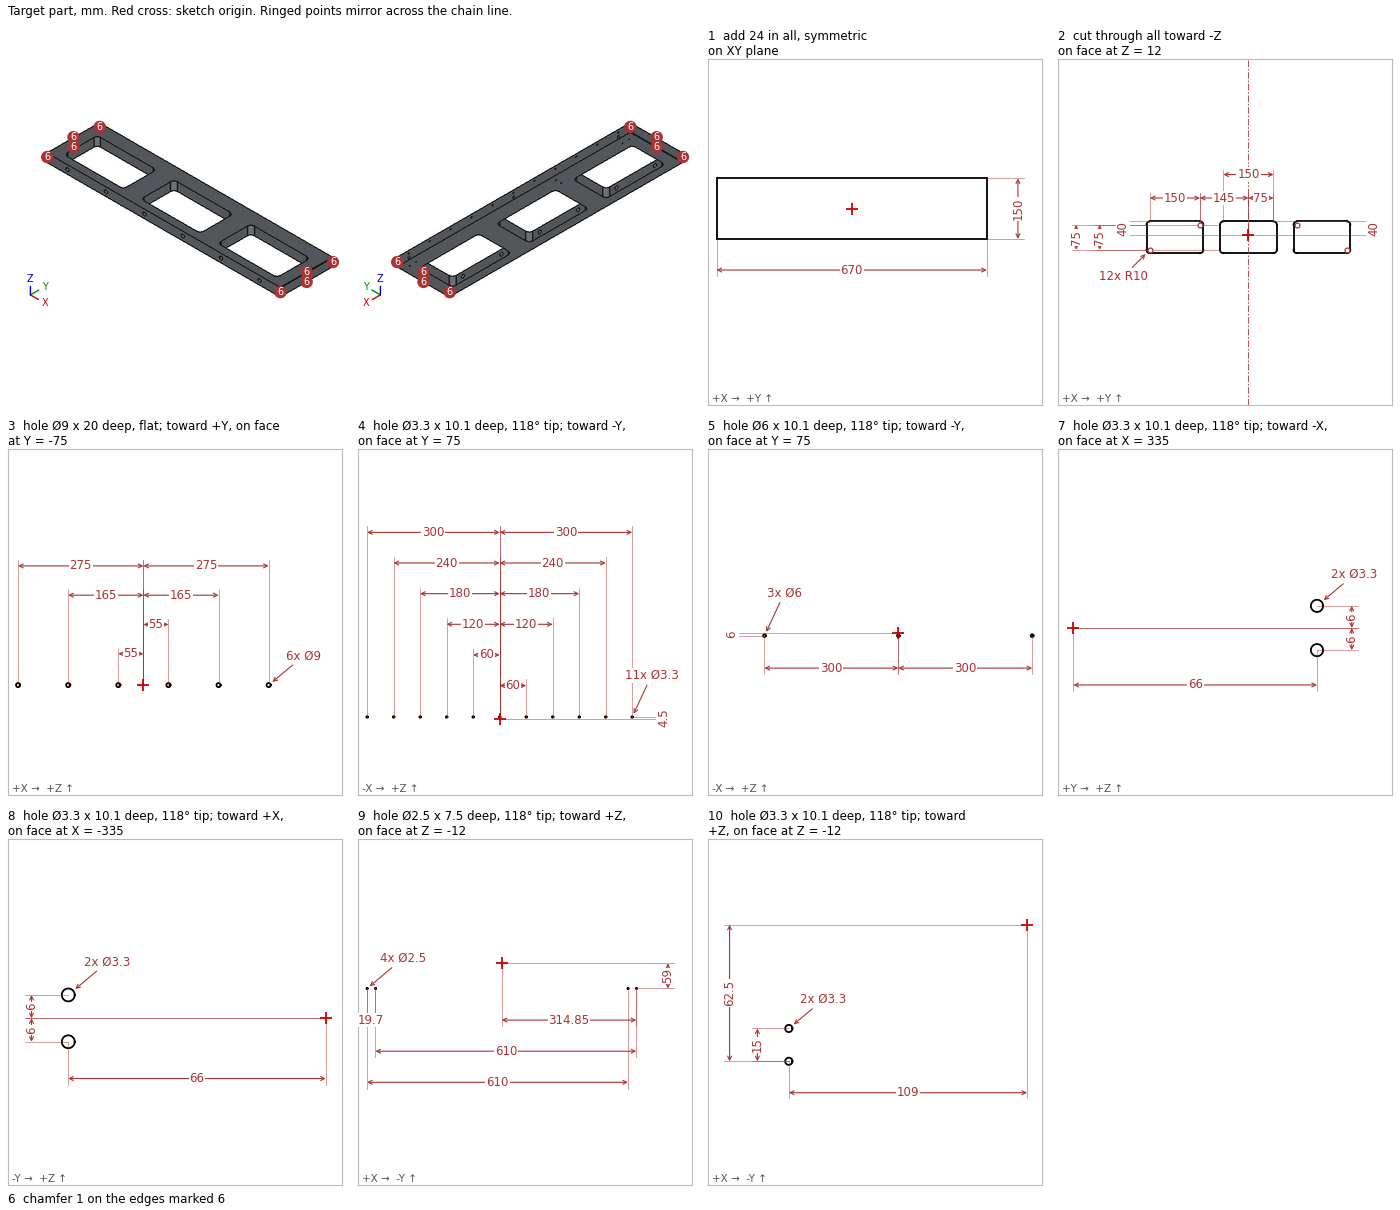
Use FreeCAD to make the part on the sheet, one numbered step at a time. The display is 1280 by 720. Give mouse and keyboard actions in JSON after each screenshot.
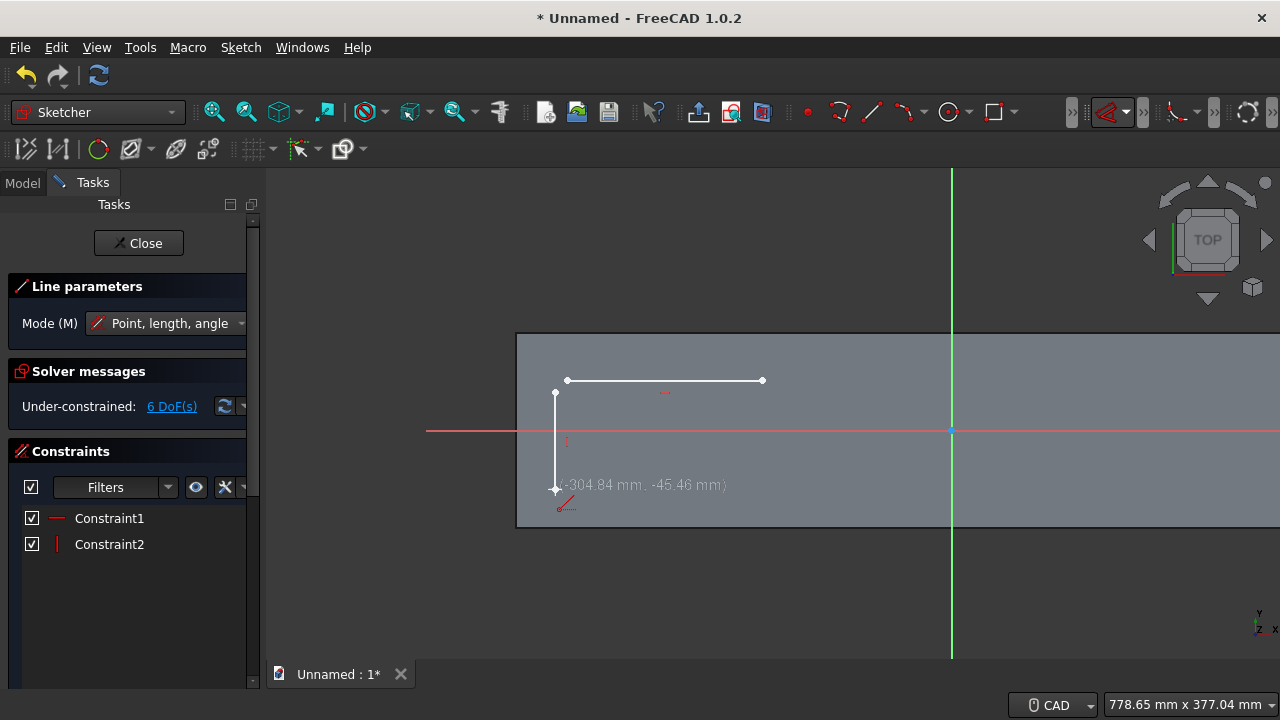
{"action": "left_click", "coordinate": [568, 502]}
{"action": "left_click", "coordinate": [763, 502]}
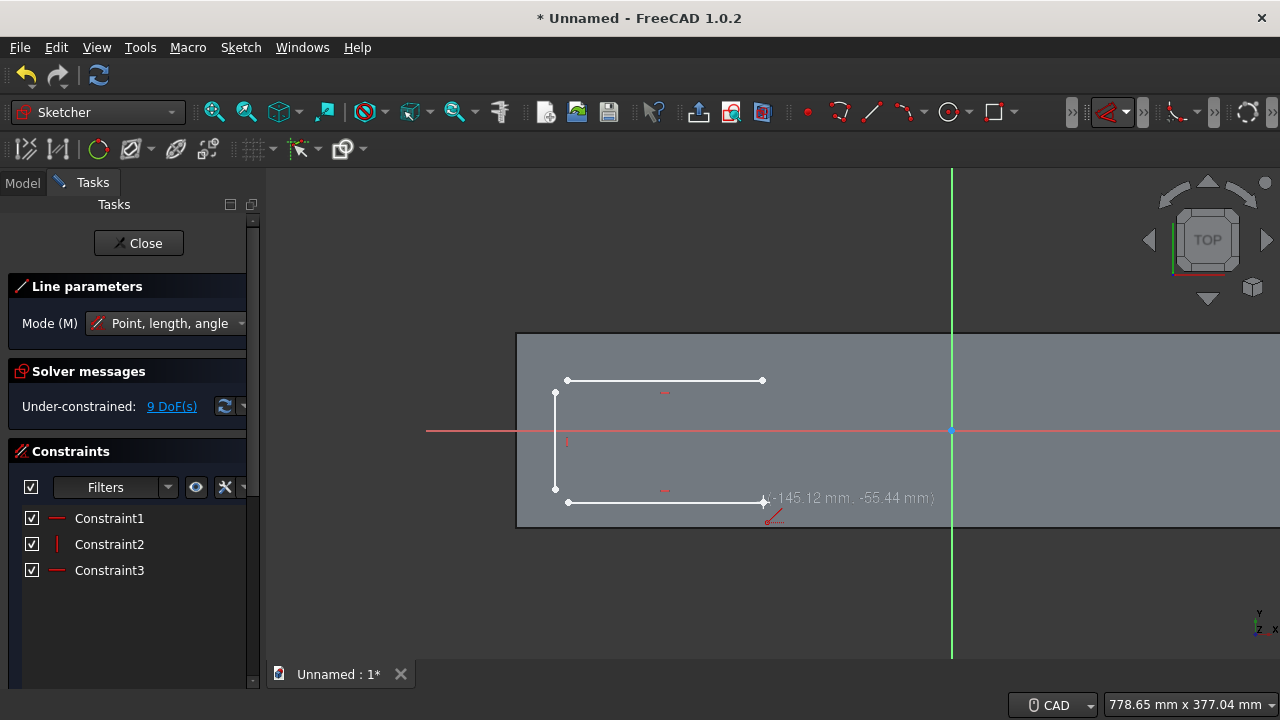
{"action": "left_click", "coordinate": [776, 489]}
{"action": "left_click", "coordinate": [776, 392]}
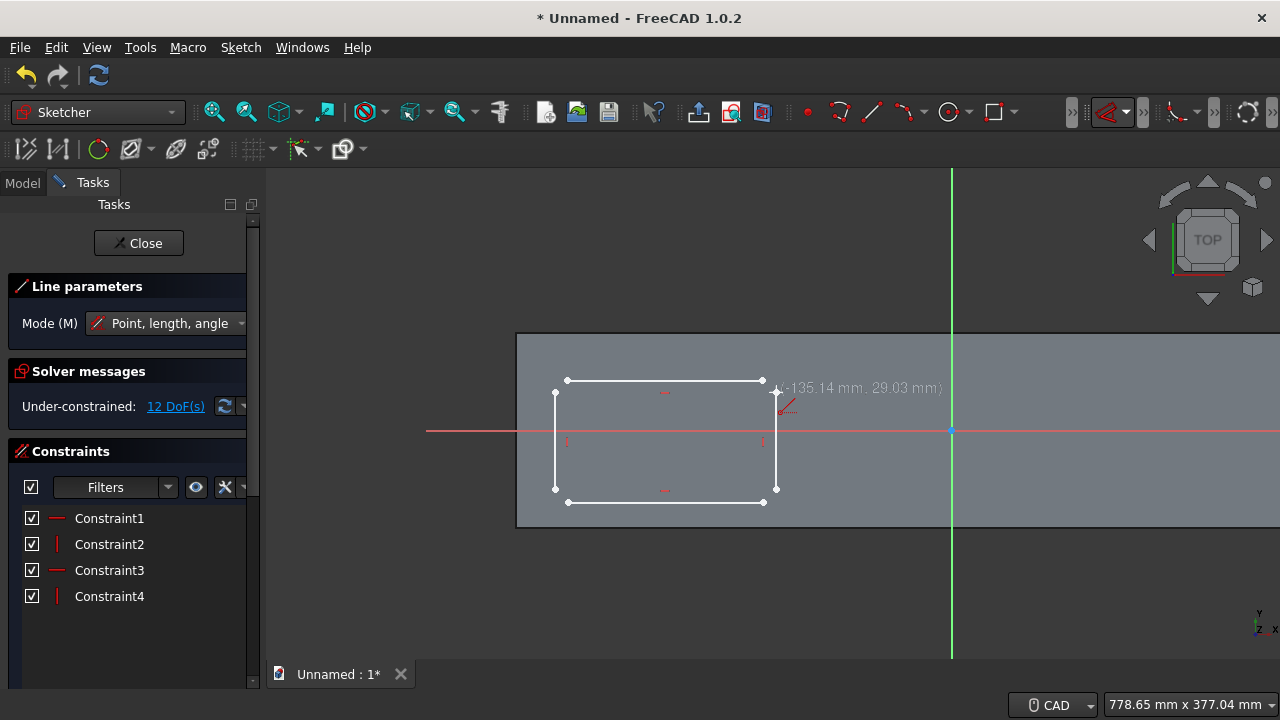
{"action": "left_click", "coordinate": [904, 112]}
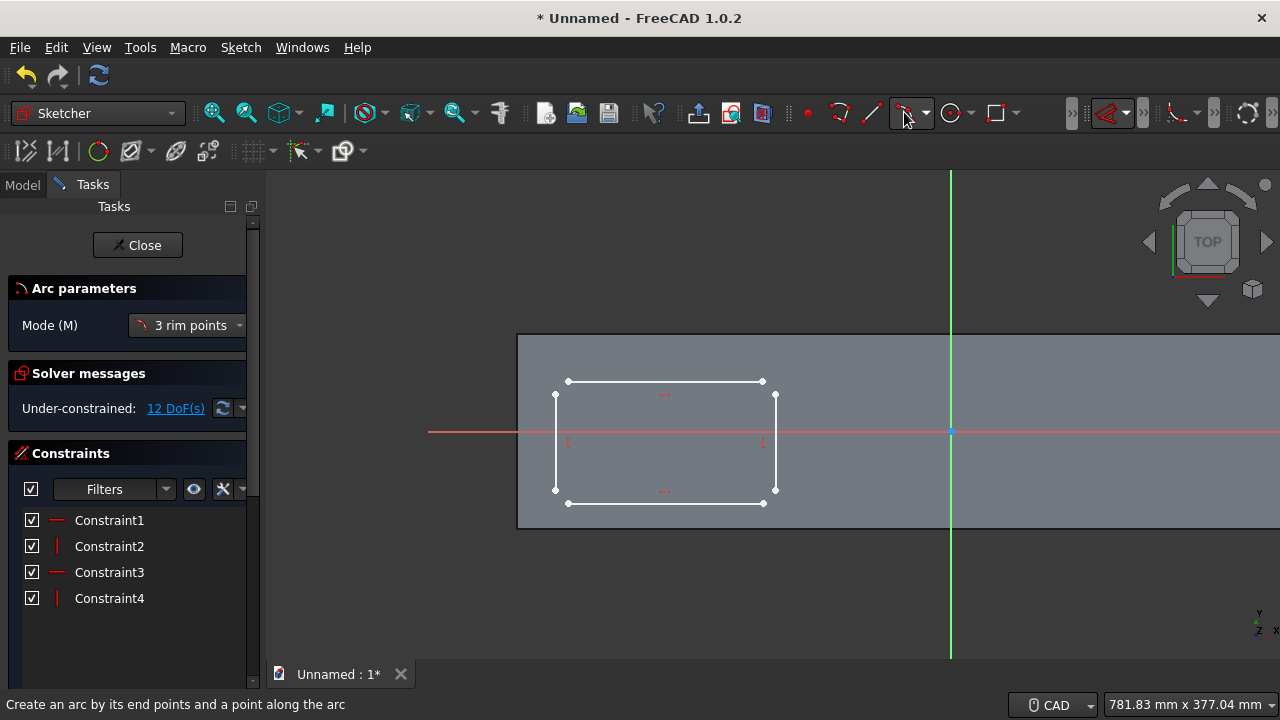
{"action": "left_click", "coordinate": [568, 382]}
{"action": "left_click", "coordinate": [556, 394]}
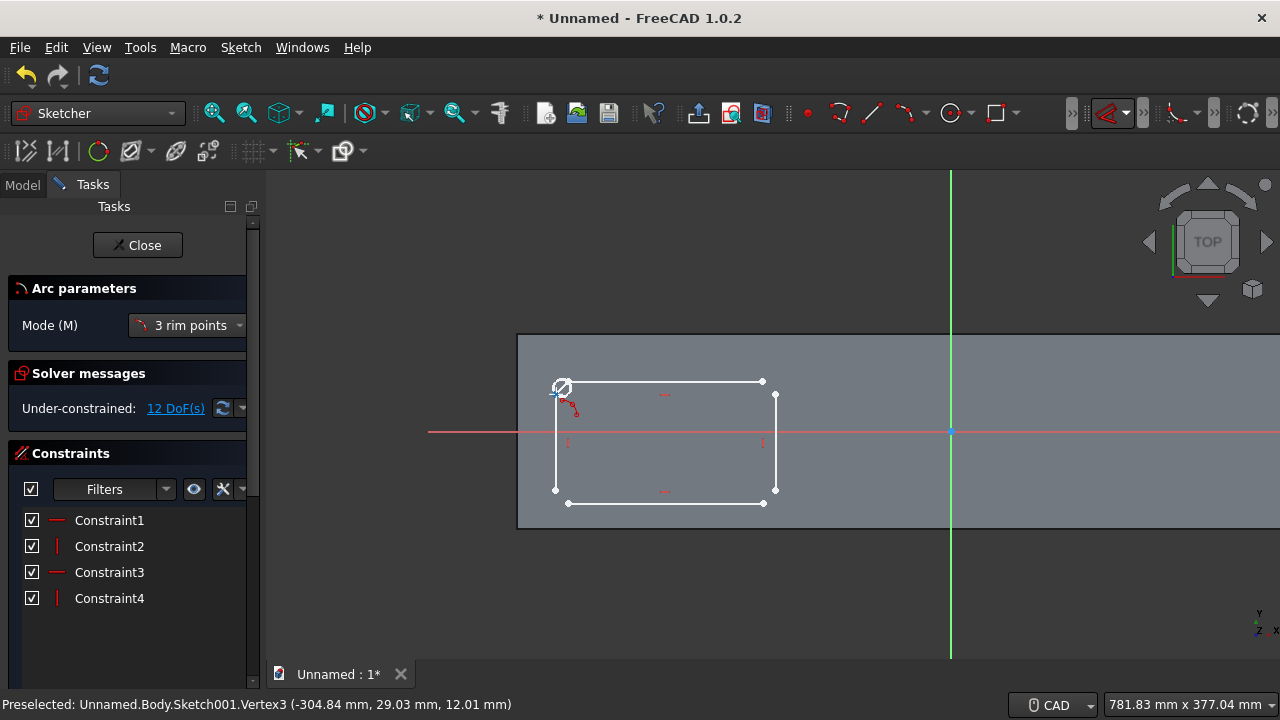
{"action": "scroll", "coordinate": [559, 384], "scroll_direction": "up", "scroll_amount": 8}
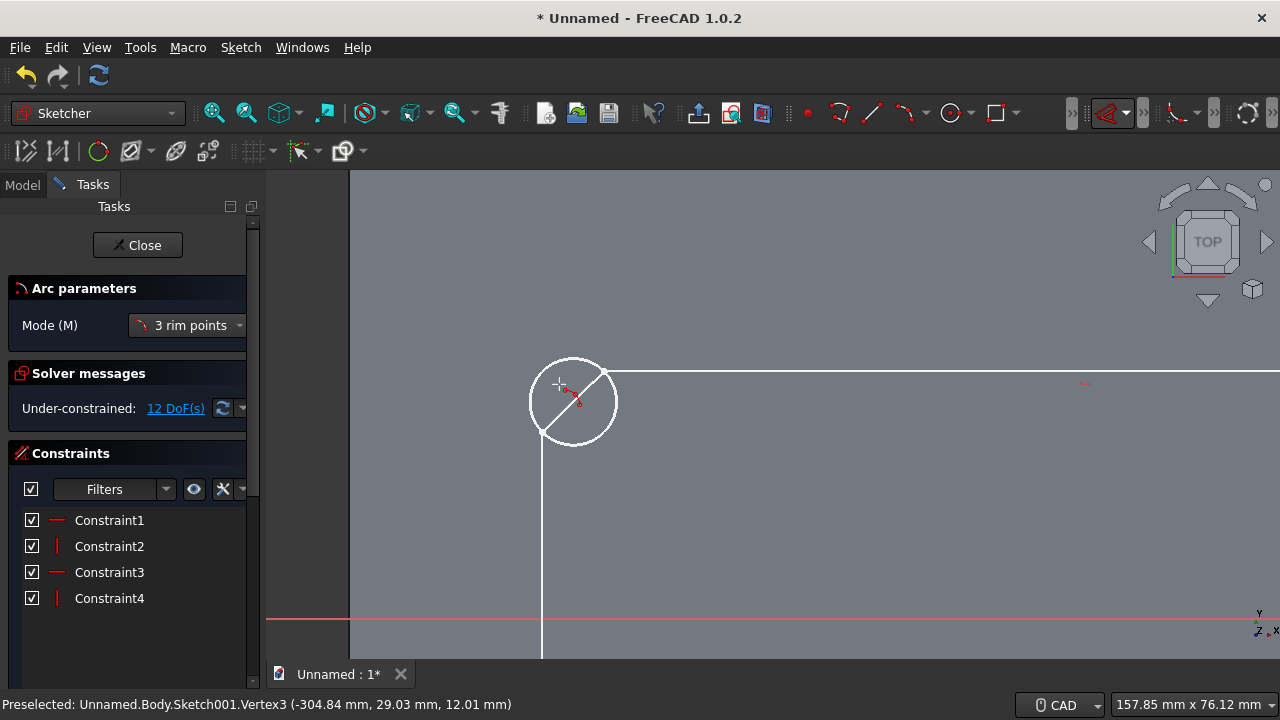
{"action": "left_click", "coordinate": [560, 381]}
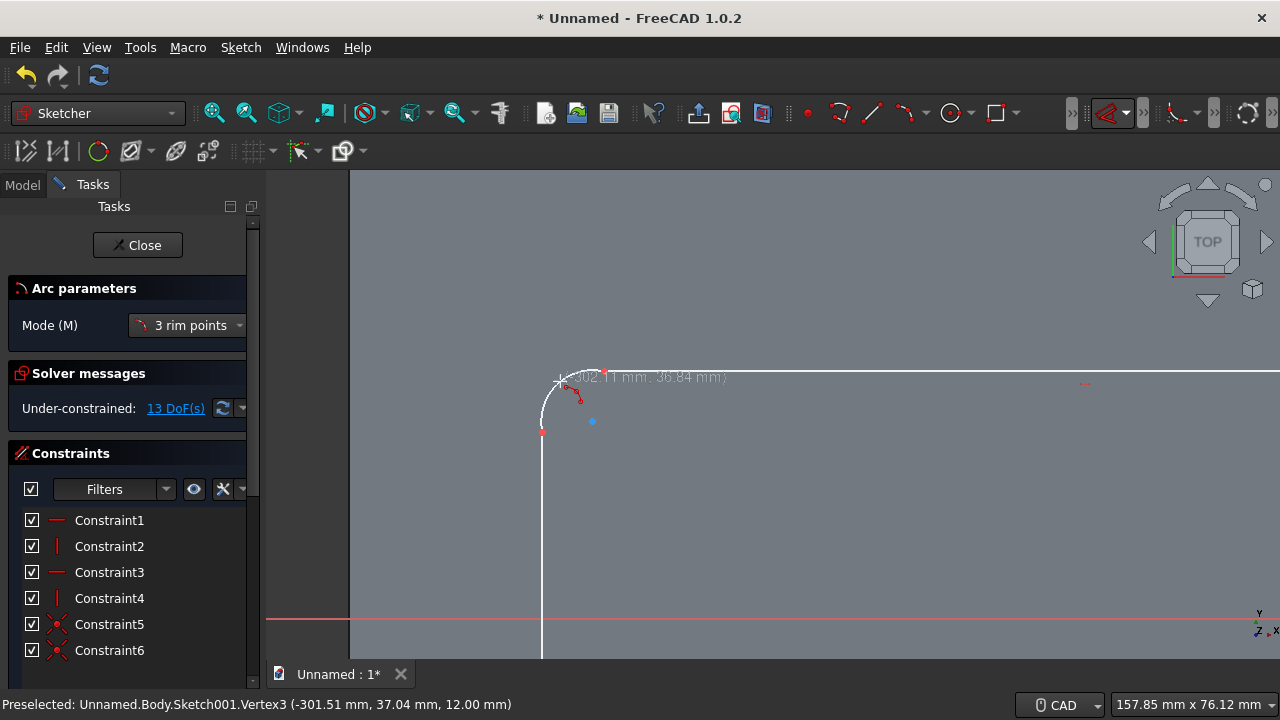
{"action": "scroll", "coordinate": [423, 375], "scroll_direction": "down", "scroll_amount": 10}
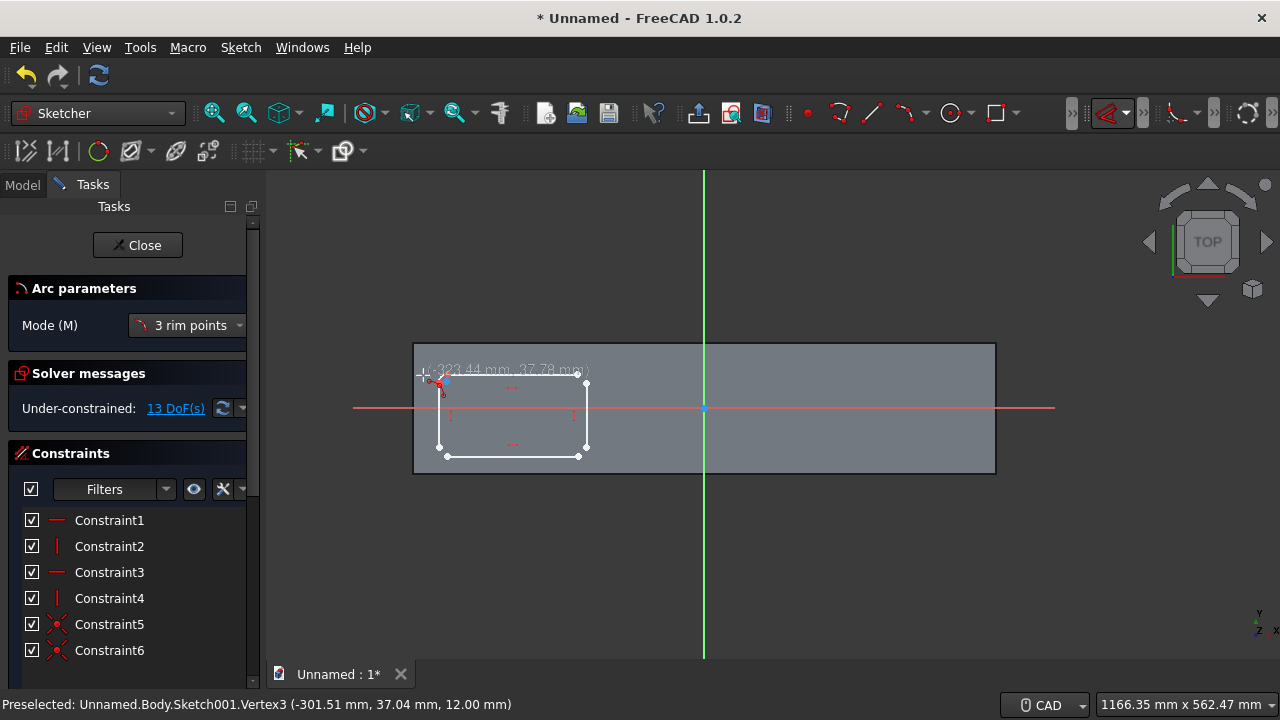
{"action": "scroll", "coordinate": [439, 447], "scroll_direction": "up", "scroll_amount": 2}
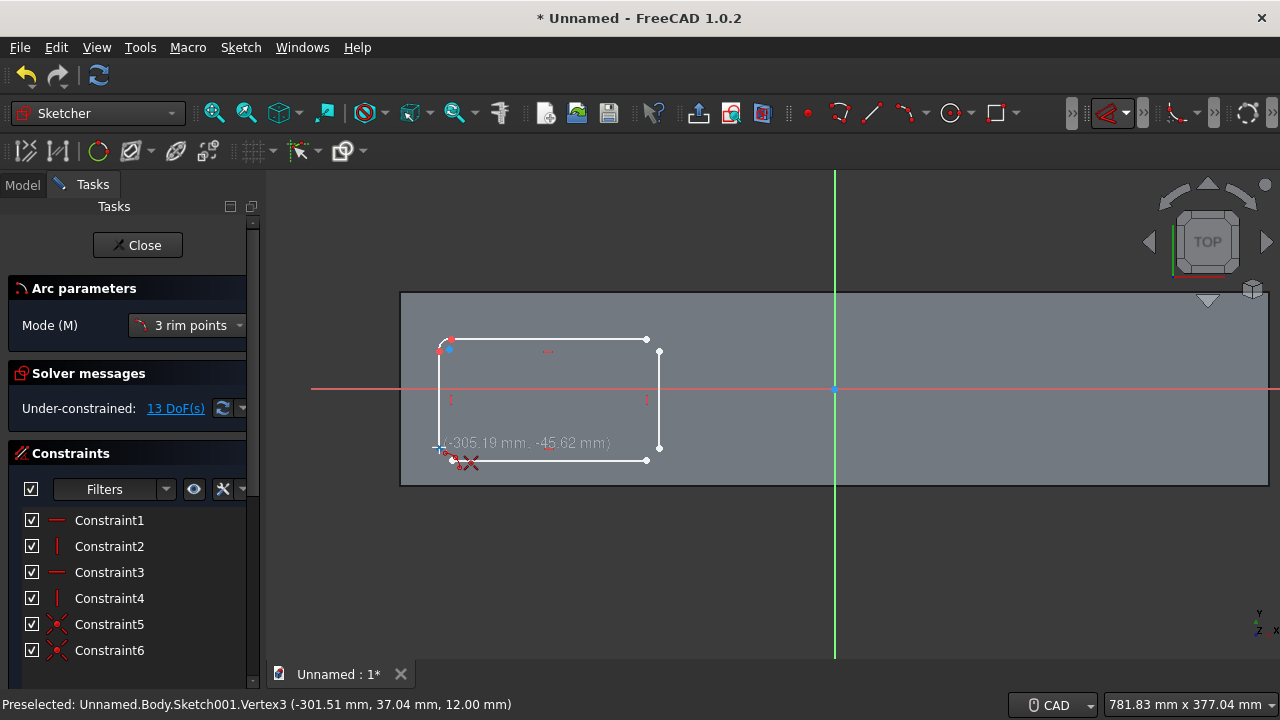
{"action": "left_click", "coordinate": [439, 448]}
{"action": "left_click", "coordinate": [452, 461]}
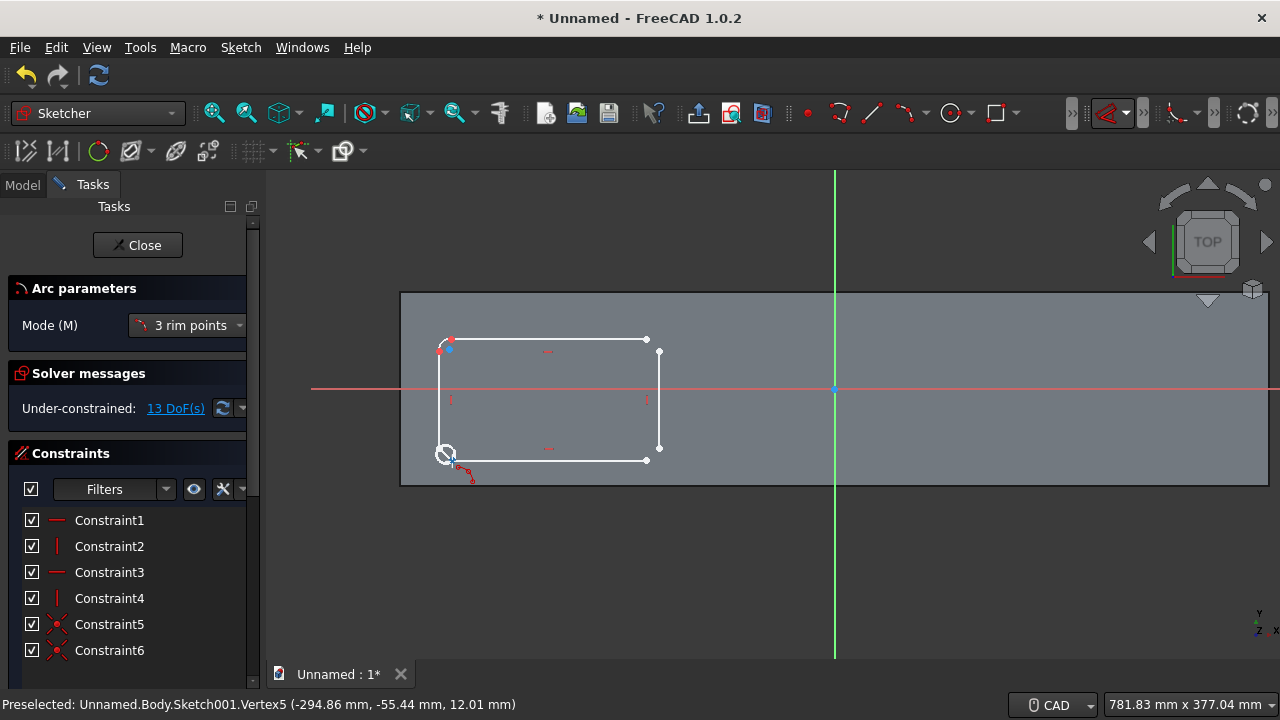
{"action": "scroll", "coordinate": [443, 457], "scroll_direction": "up", "scroll_amount": 8}